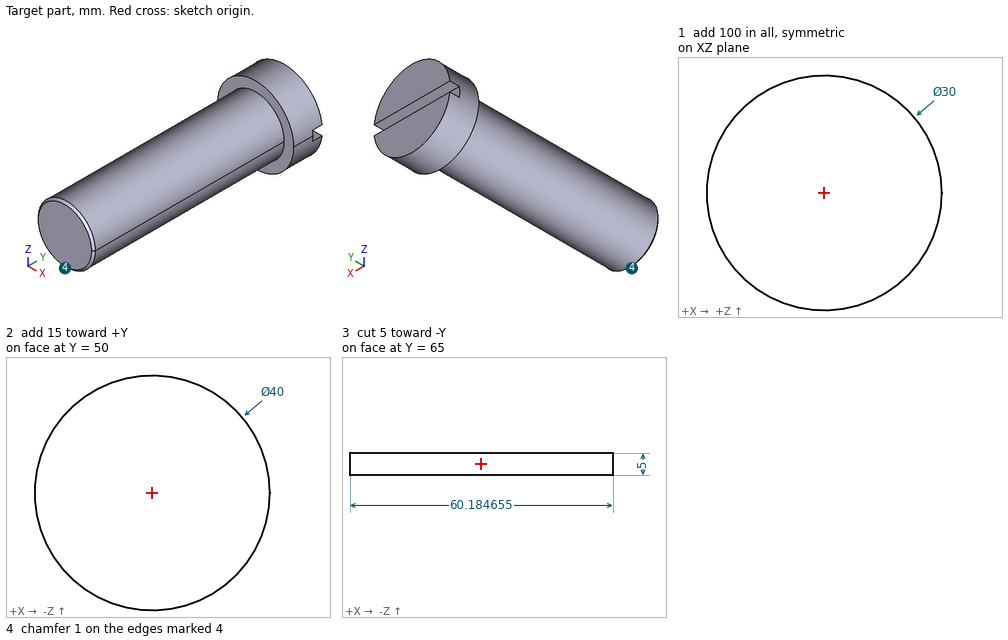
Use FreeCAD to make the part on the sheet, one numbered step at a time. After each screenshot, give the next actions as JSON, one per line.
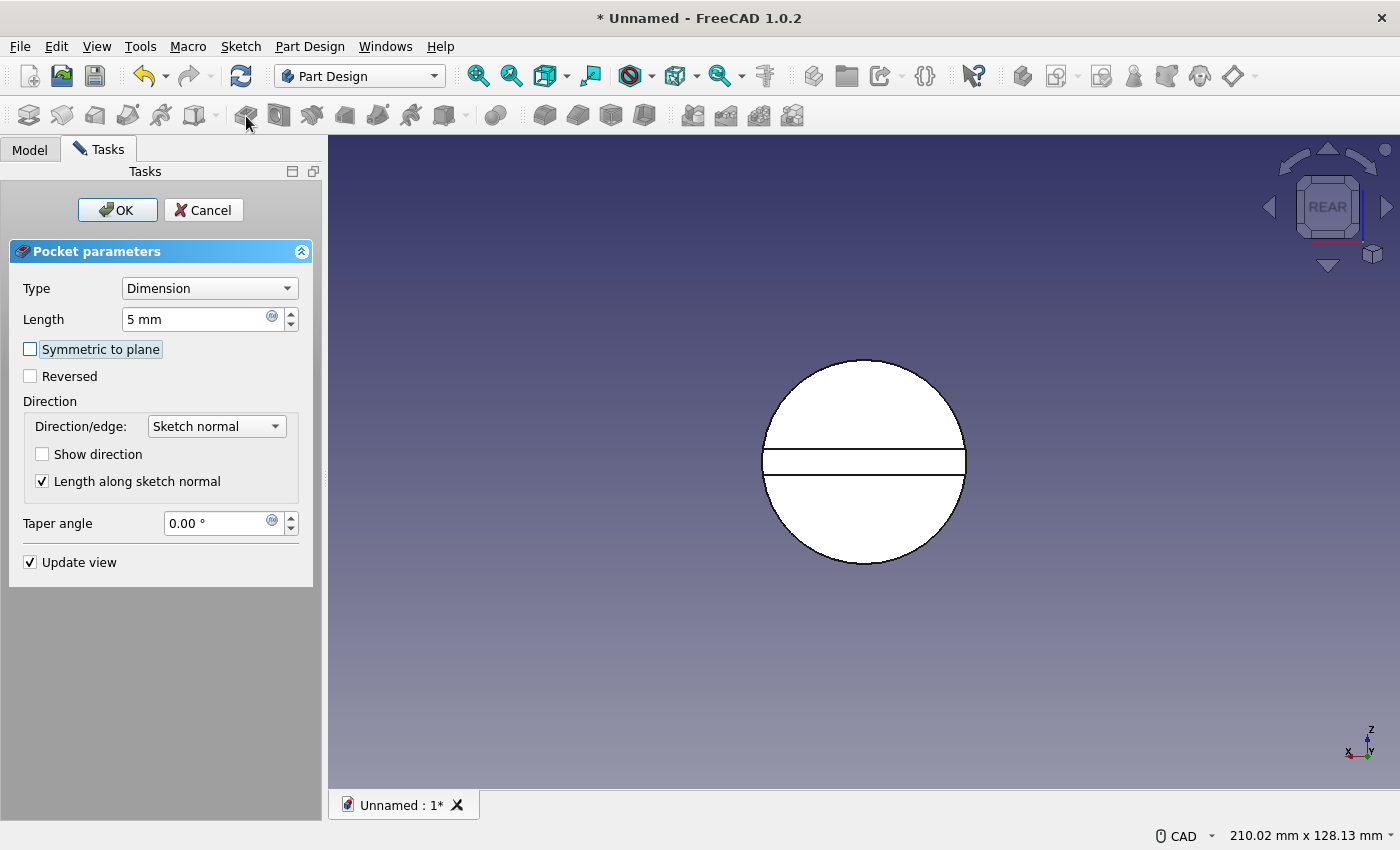
{"action": "left_click", "coordinate": [118, 210]}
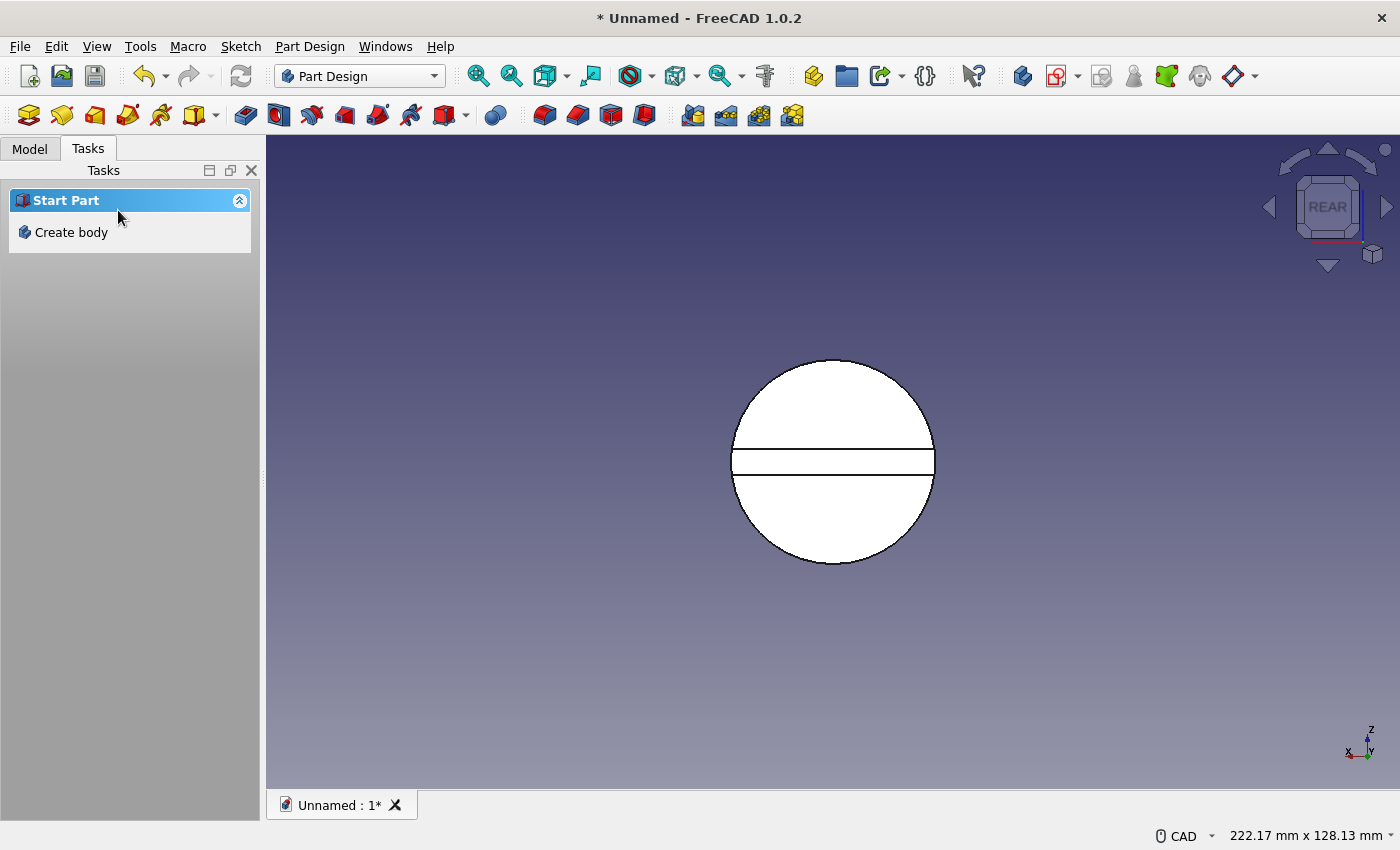
{"action": "left_click", "coordinate": [479, 76]}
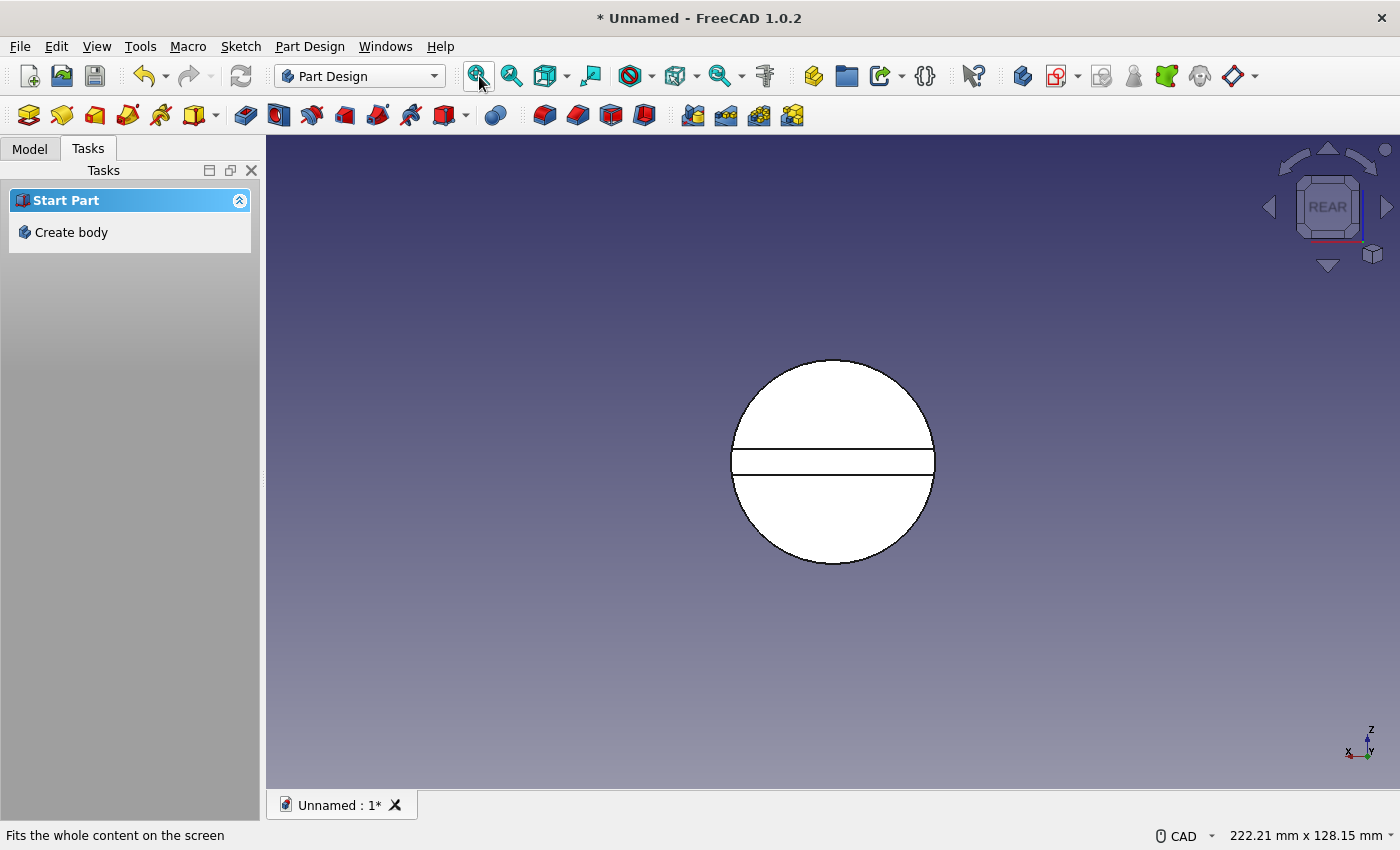
{"action": "key", "text": "0"}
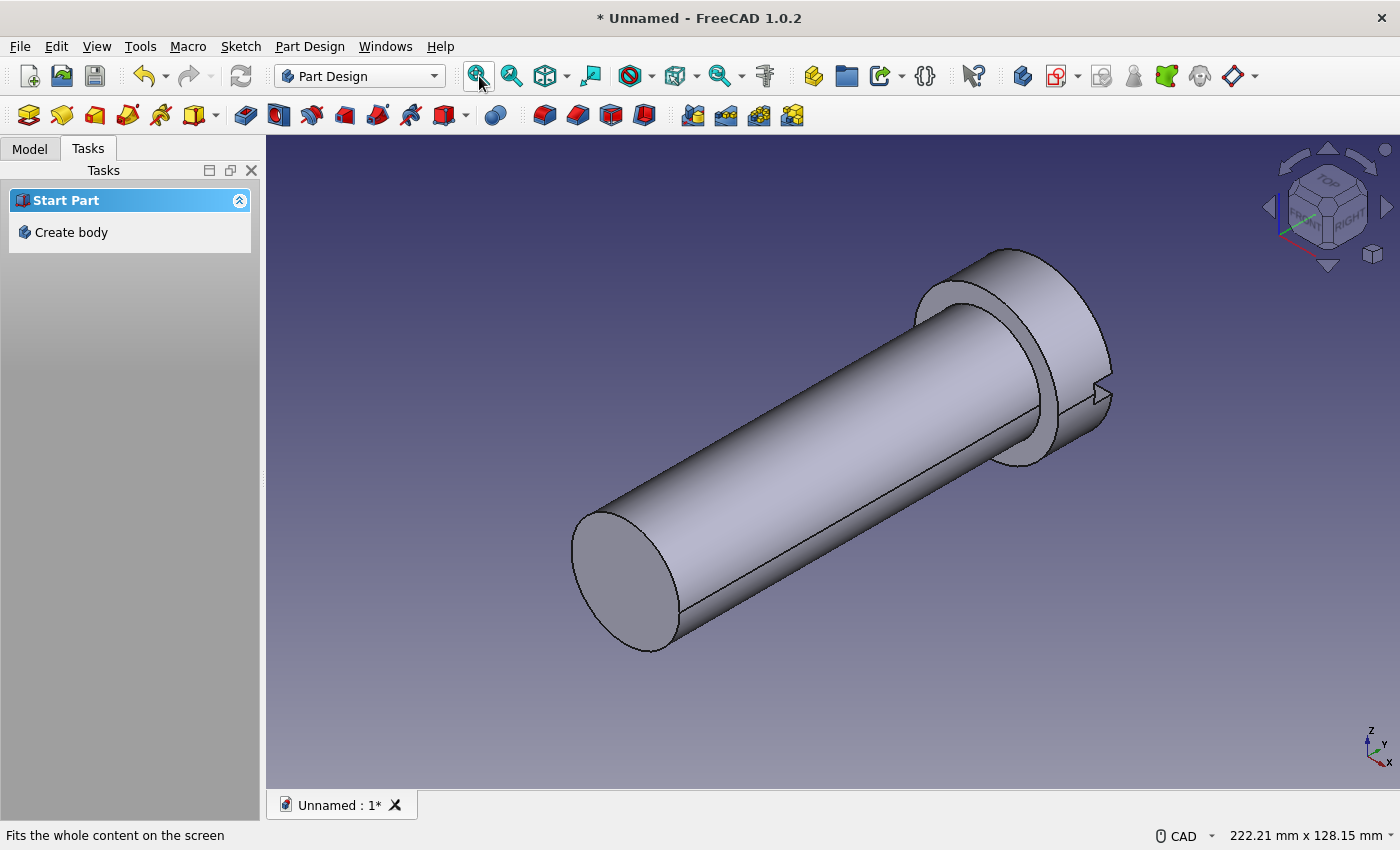
{"action": "left_click", "coordinate": [609, 512]}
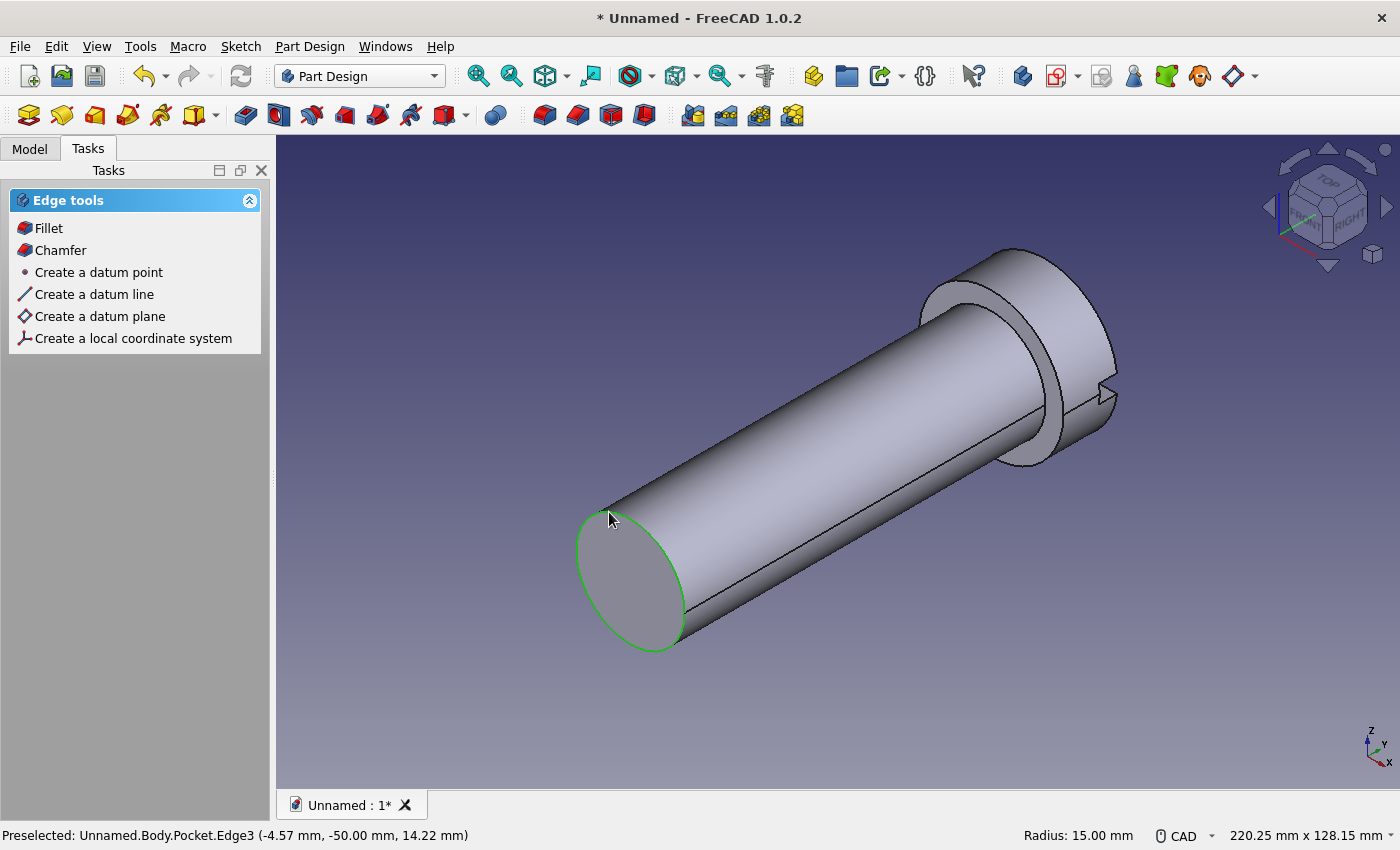
{"action": "left_click", "coordinate": [578, 116]}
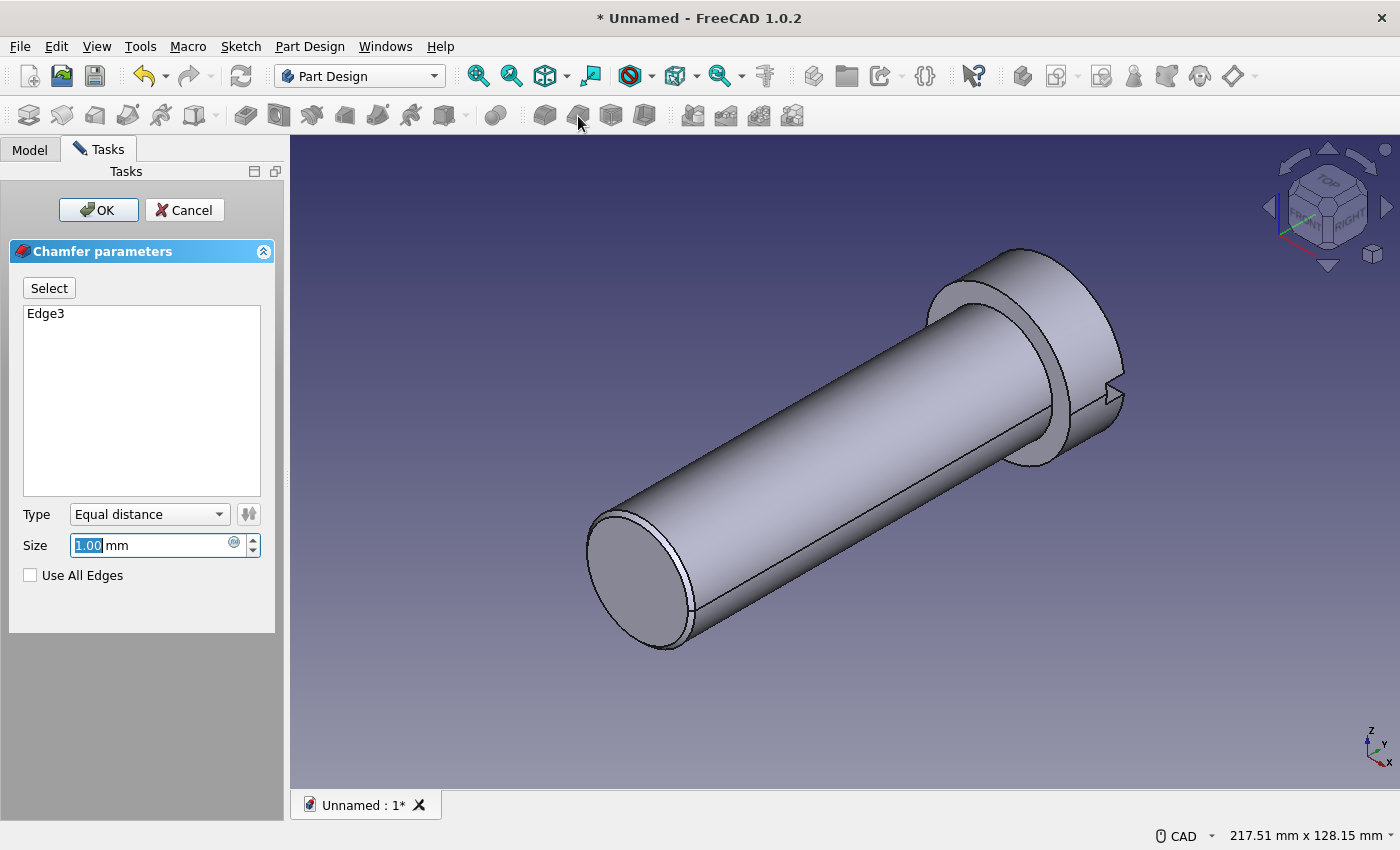
{"action": "type", "text": "1"}
{"action": "key", "text": "Tab"}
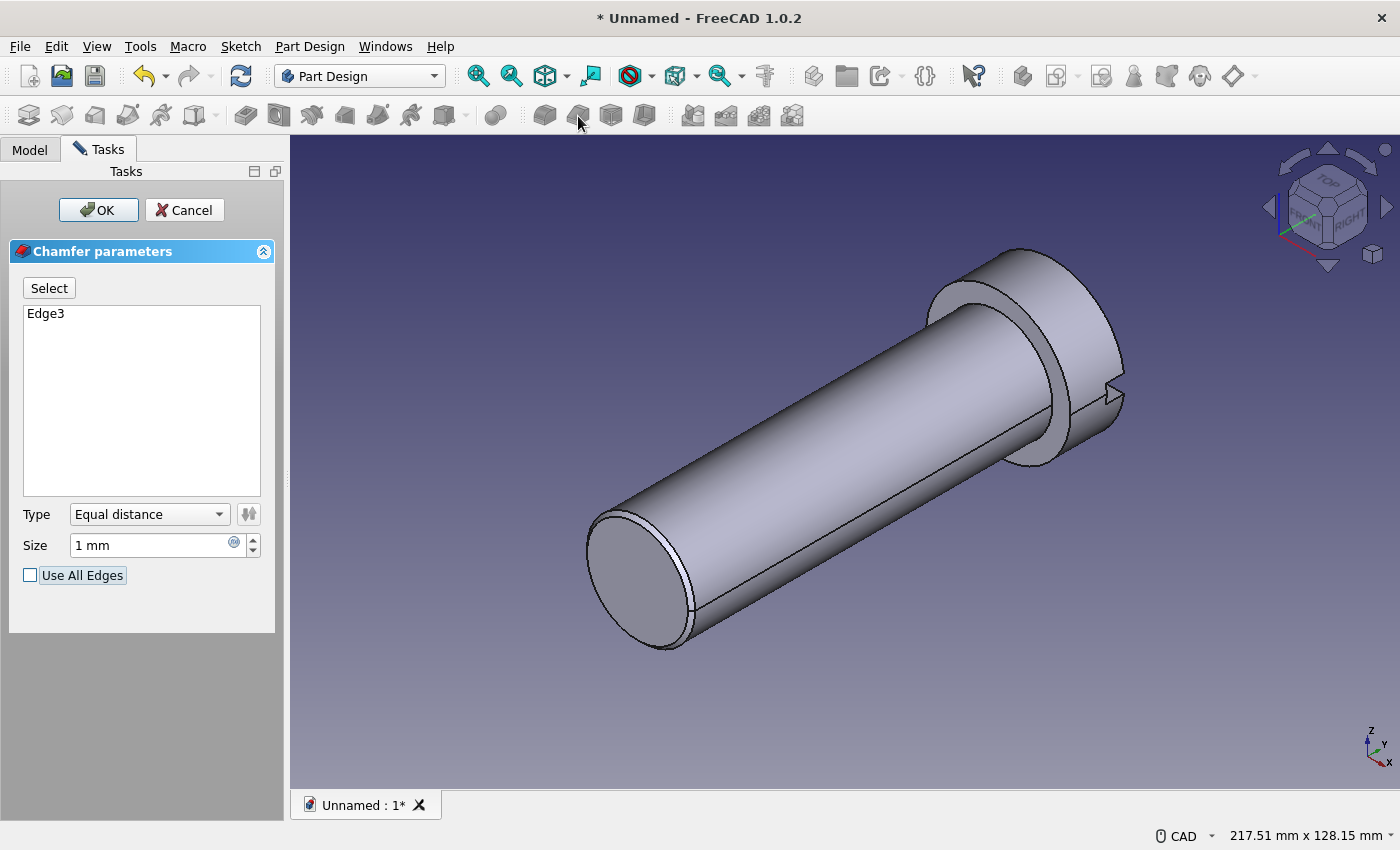
{"action": "left_click", "coordinate": [99, 210]}